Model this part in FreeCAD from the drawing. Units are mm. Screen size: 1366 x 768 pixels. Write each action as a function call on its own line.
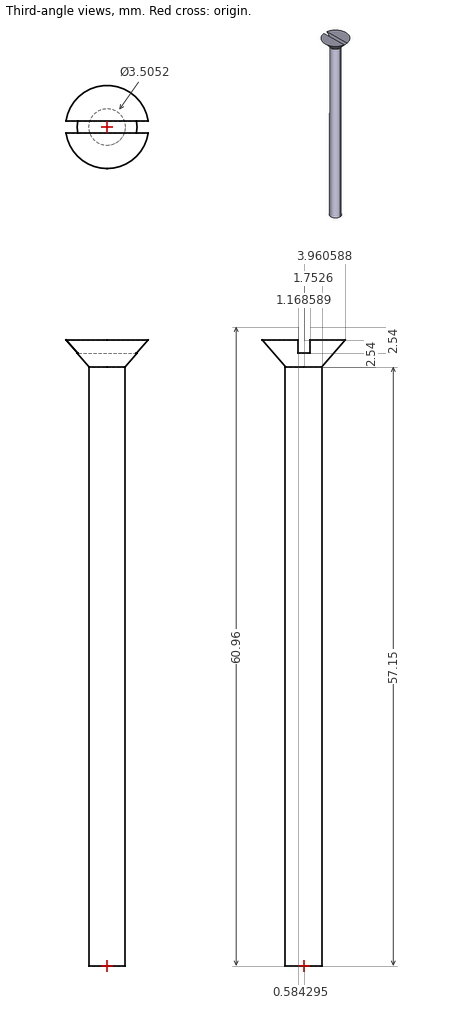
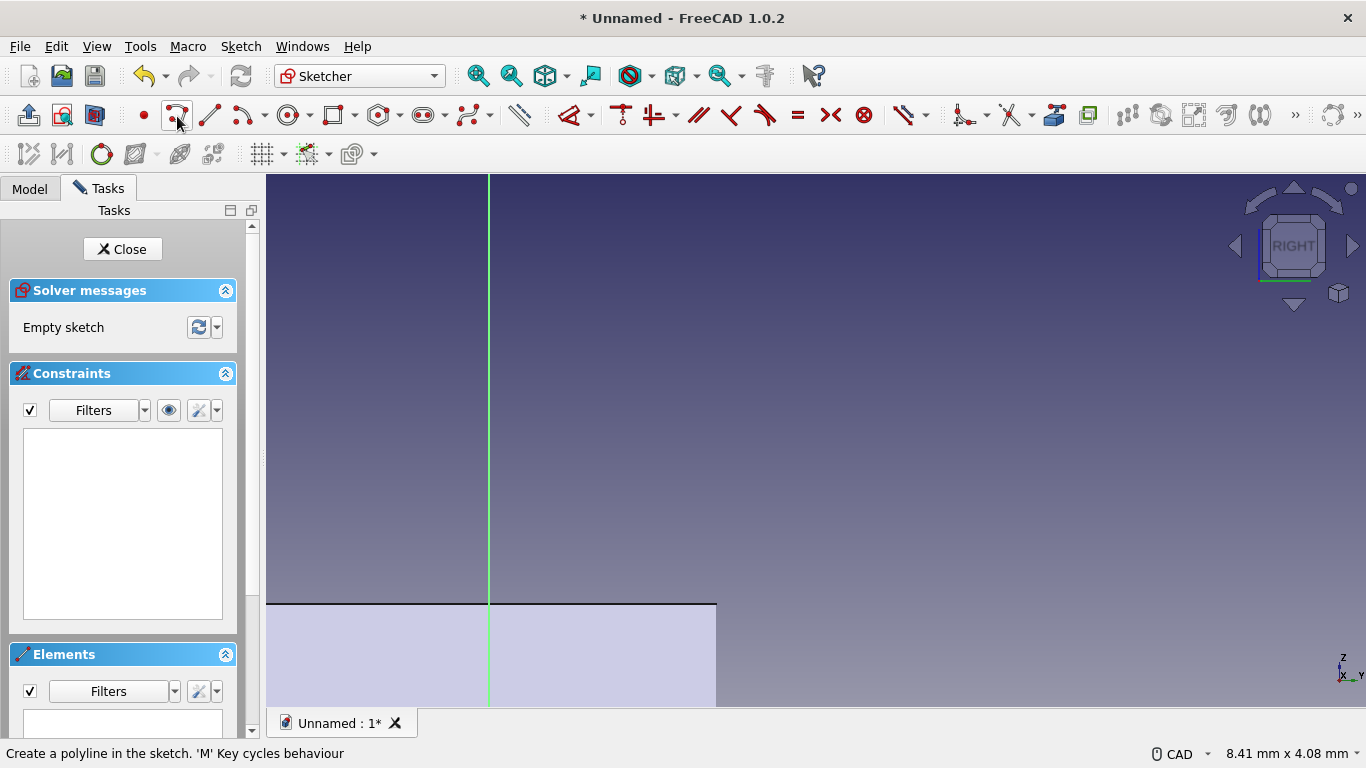
click(489, 604)
click(718, 604)
click(1006, 272)
click(498, 272)
click(489, 605)
key(Escape)
key(Escape)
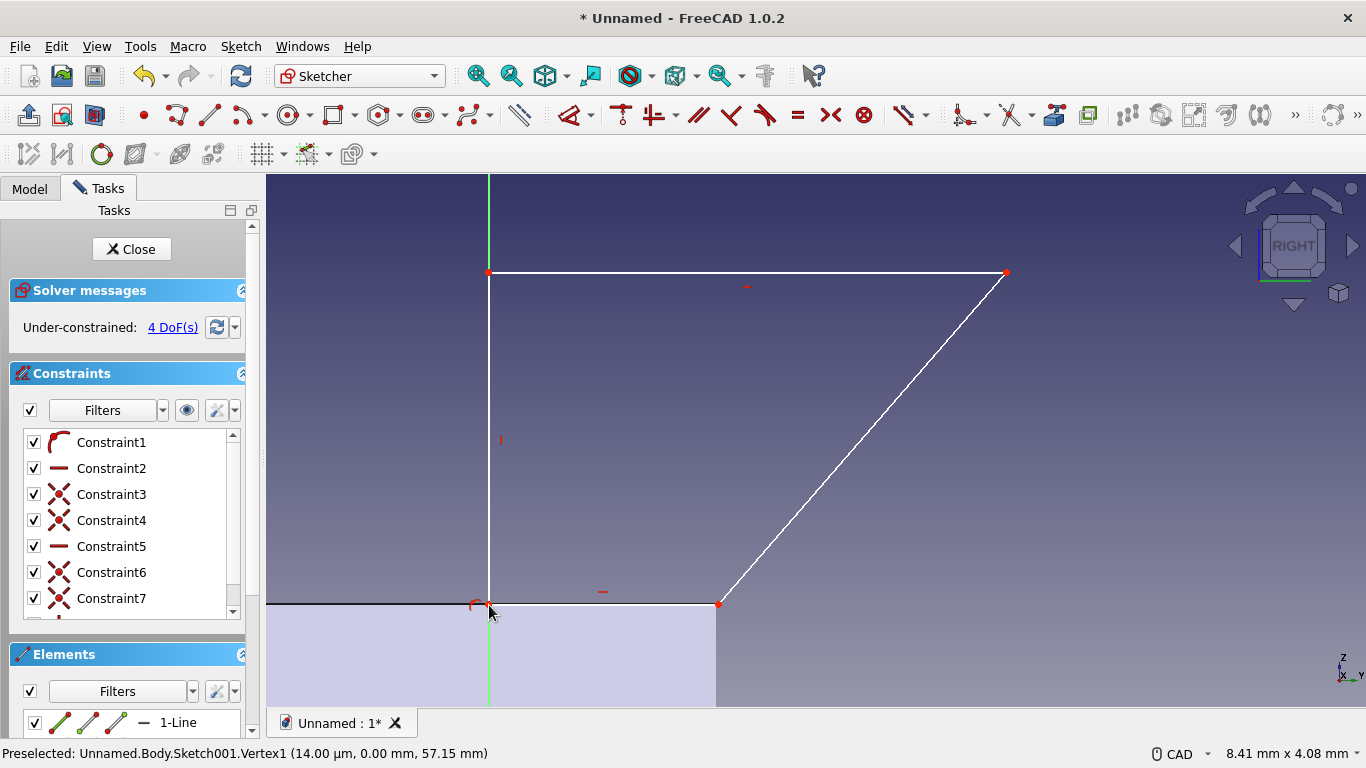
click(568, 116)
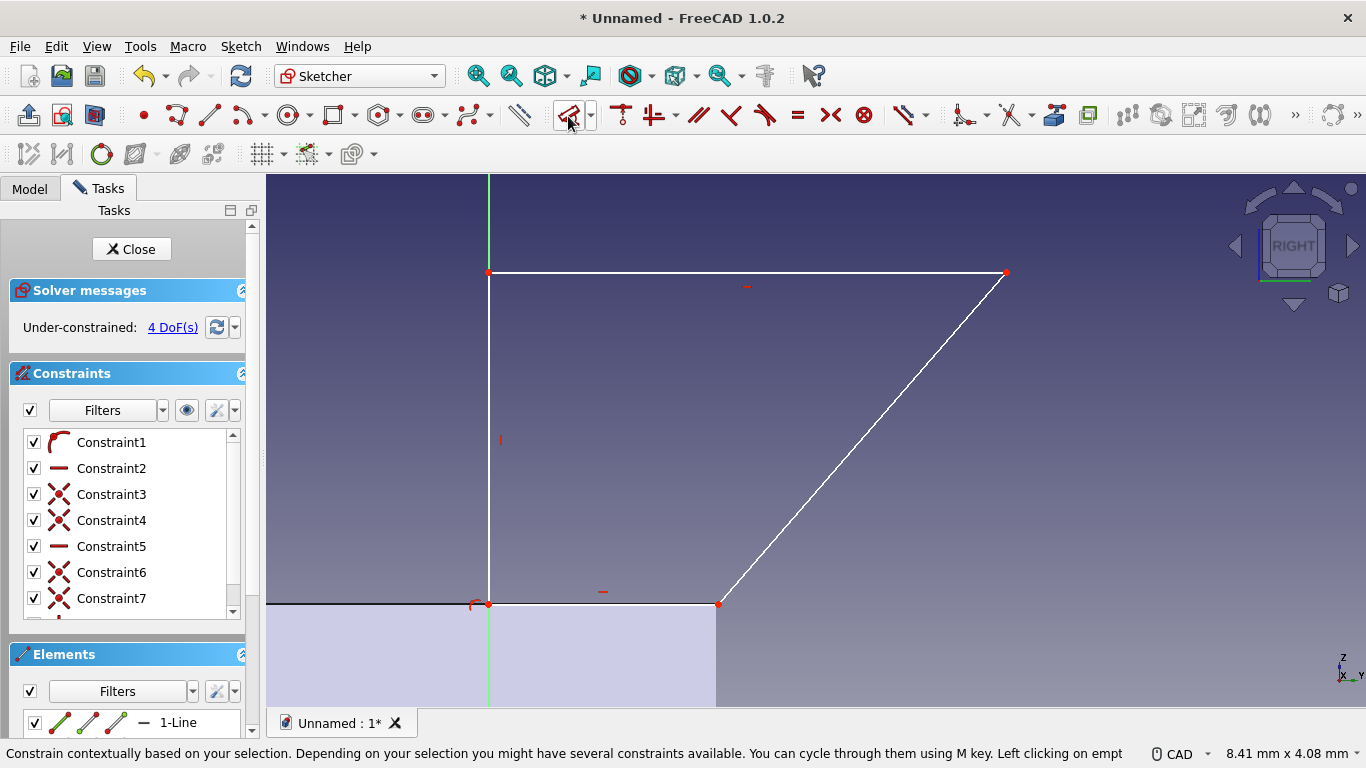
click(489, 373)
click(455, 439)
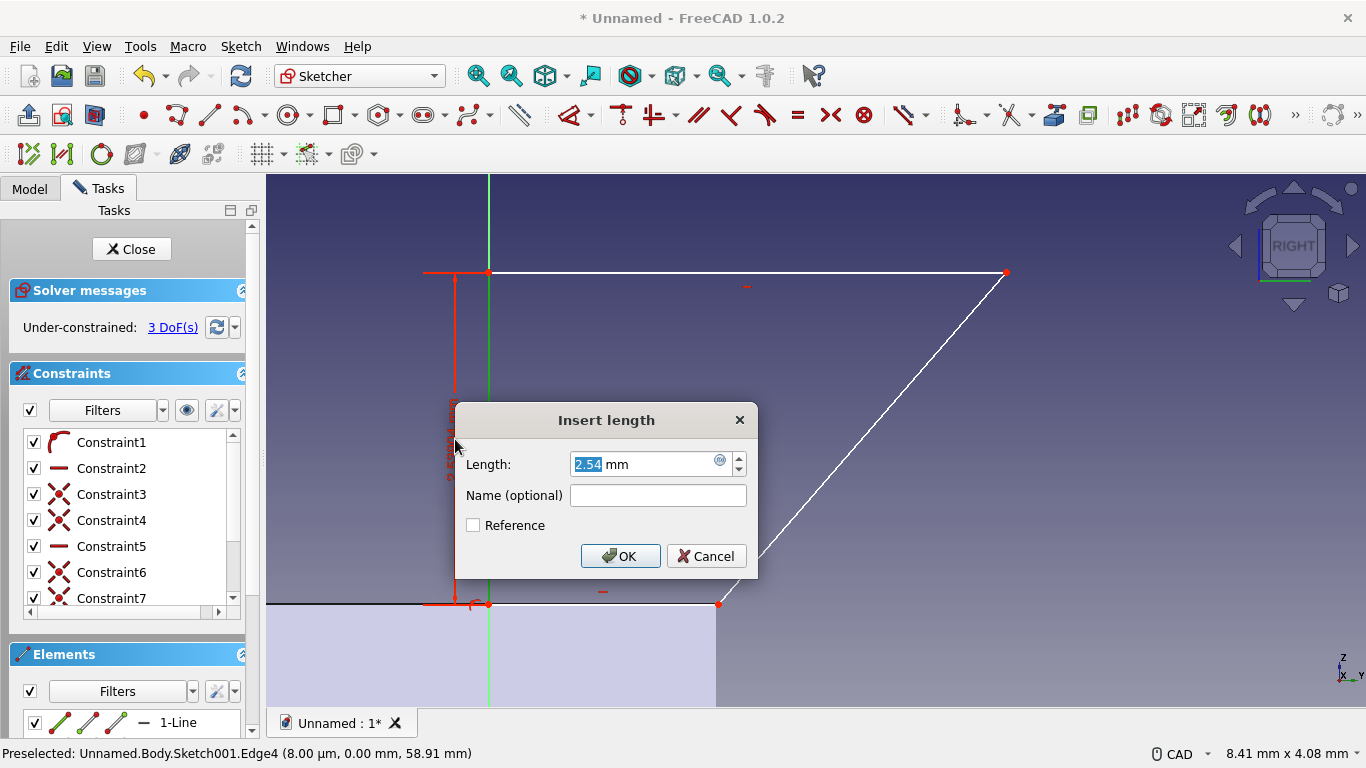
text(2.54)
key(Return)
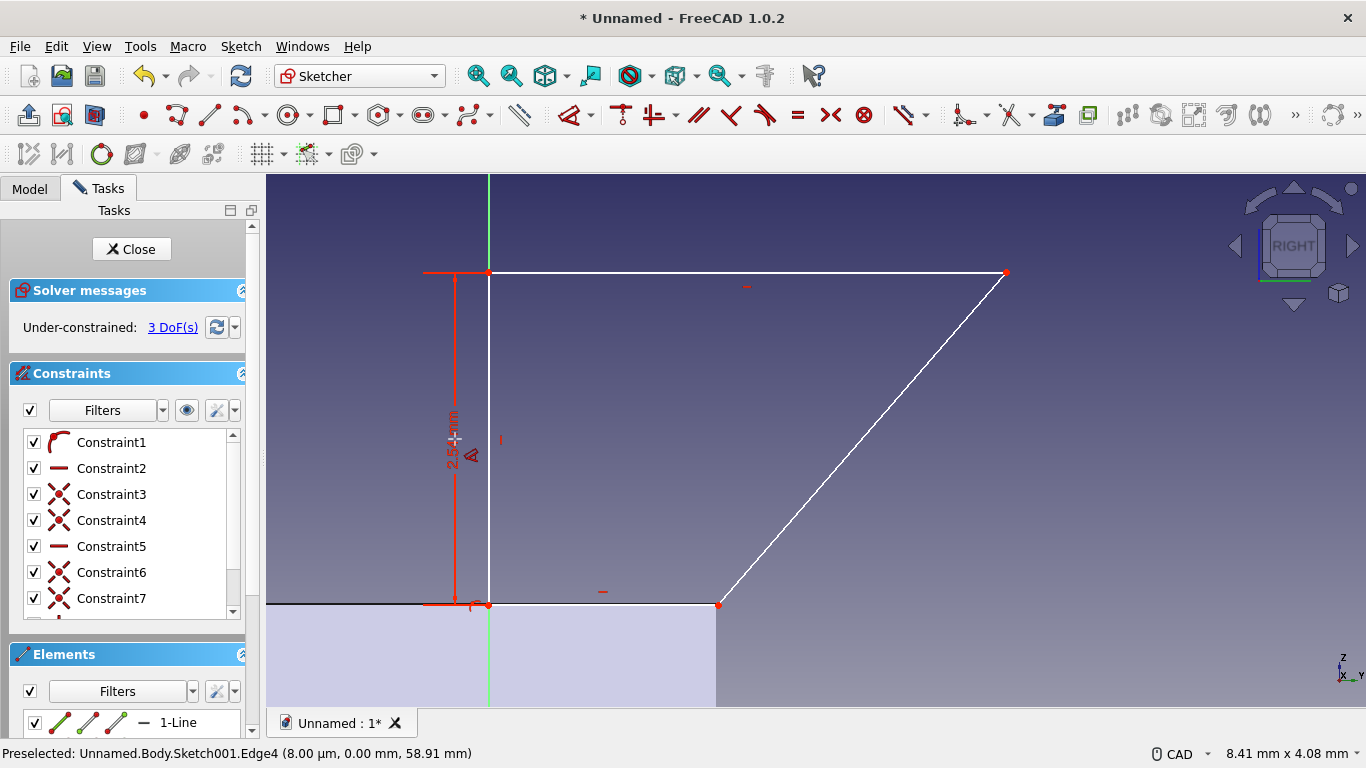
click(557, 605)
click(603, 639)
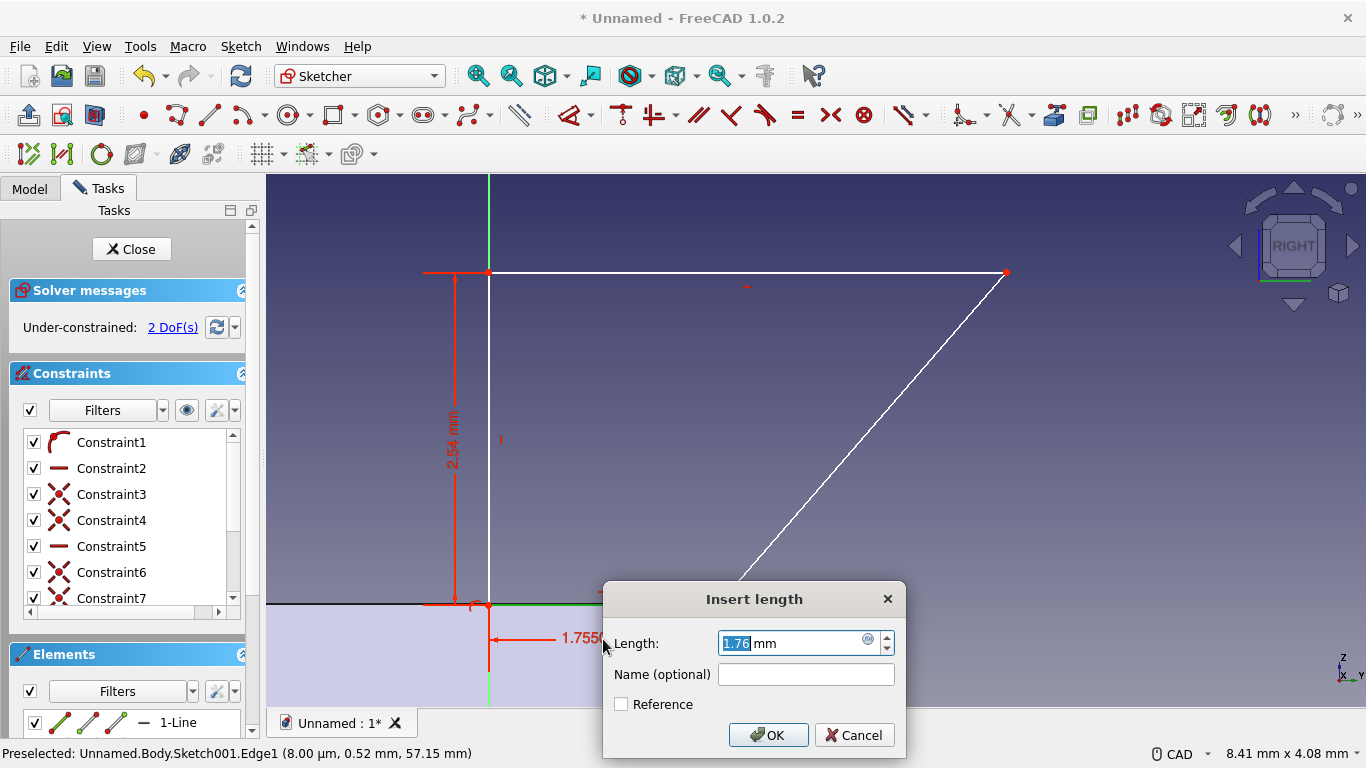
text(1.7526)
key(Return)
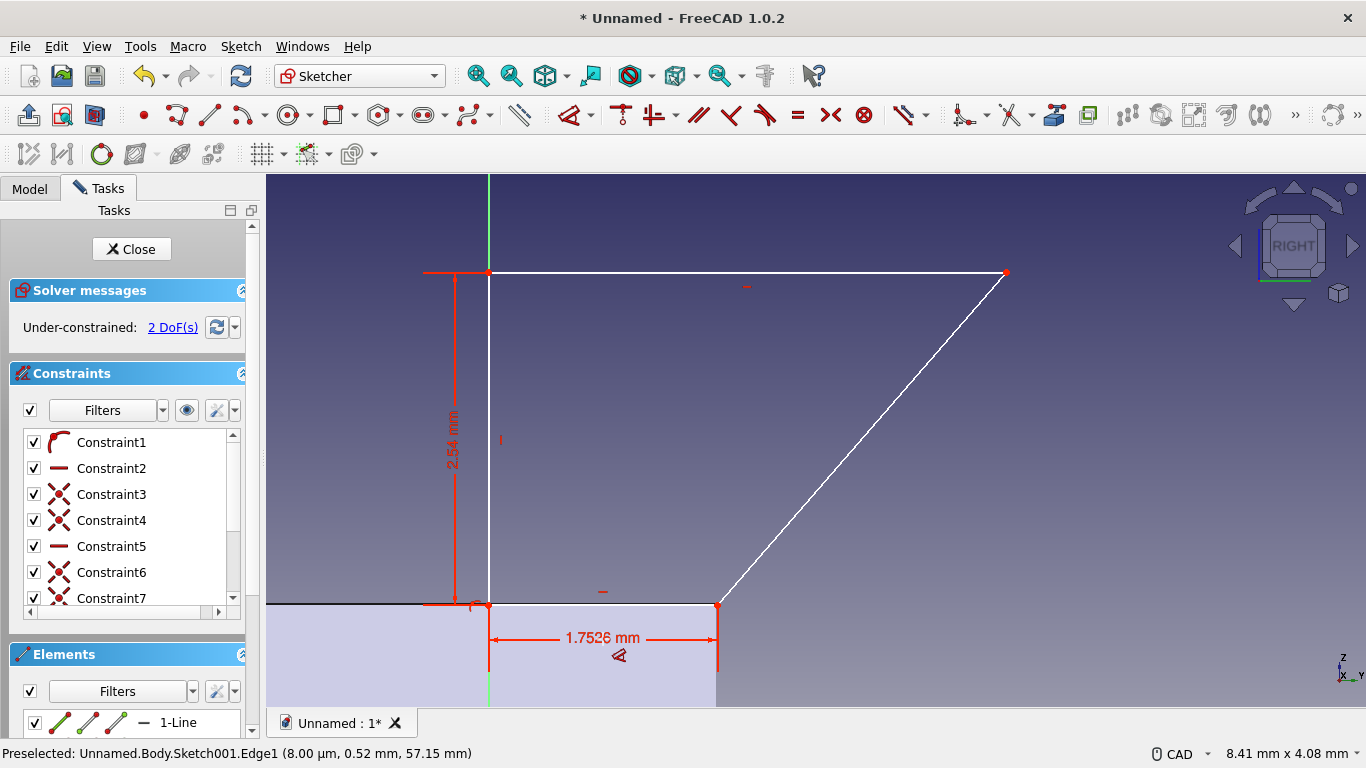
click(489, 605)
click(455, 642)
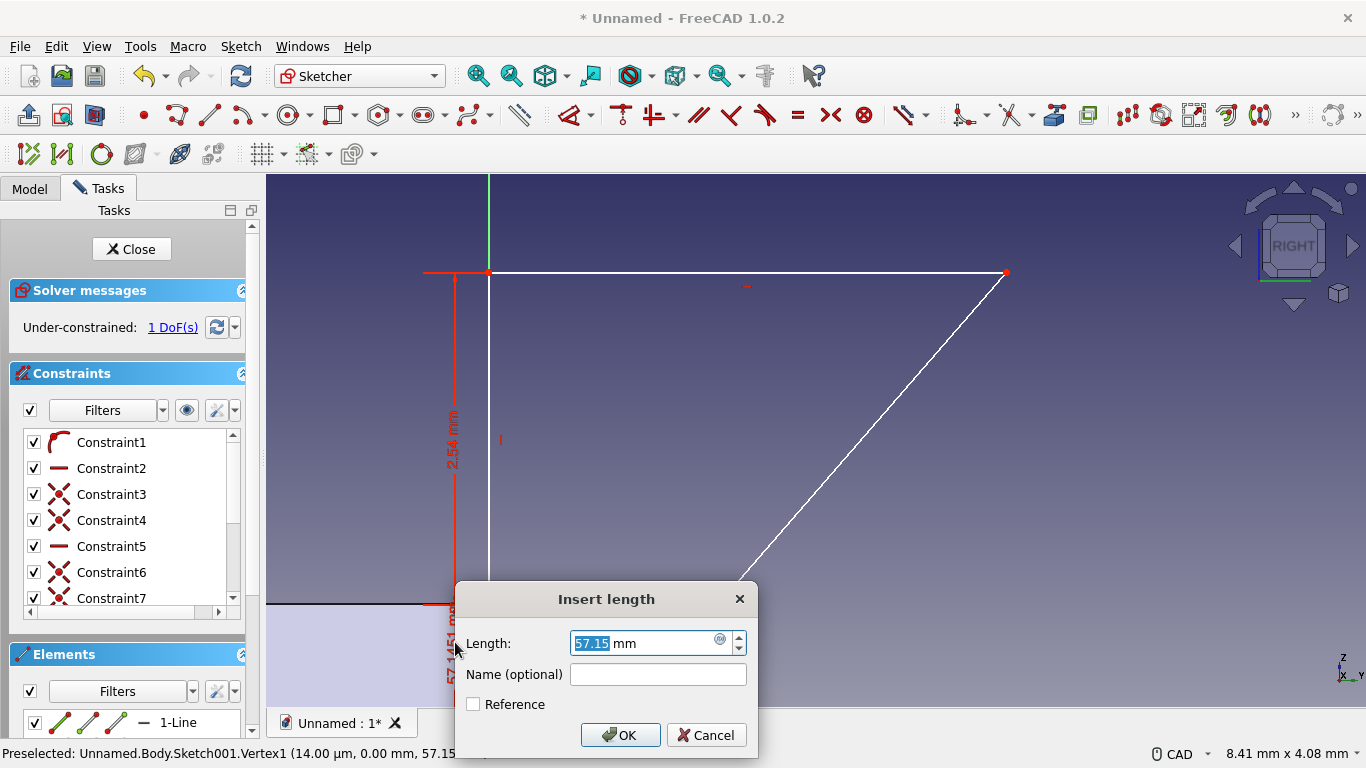
text(57.15)
key(Return)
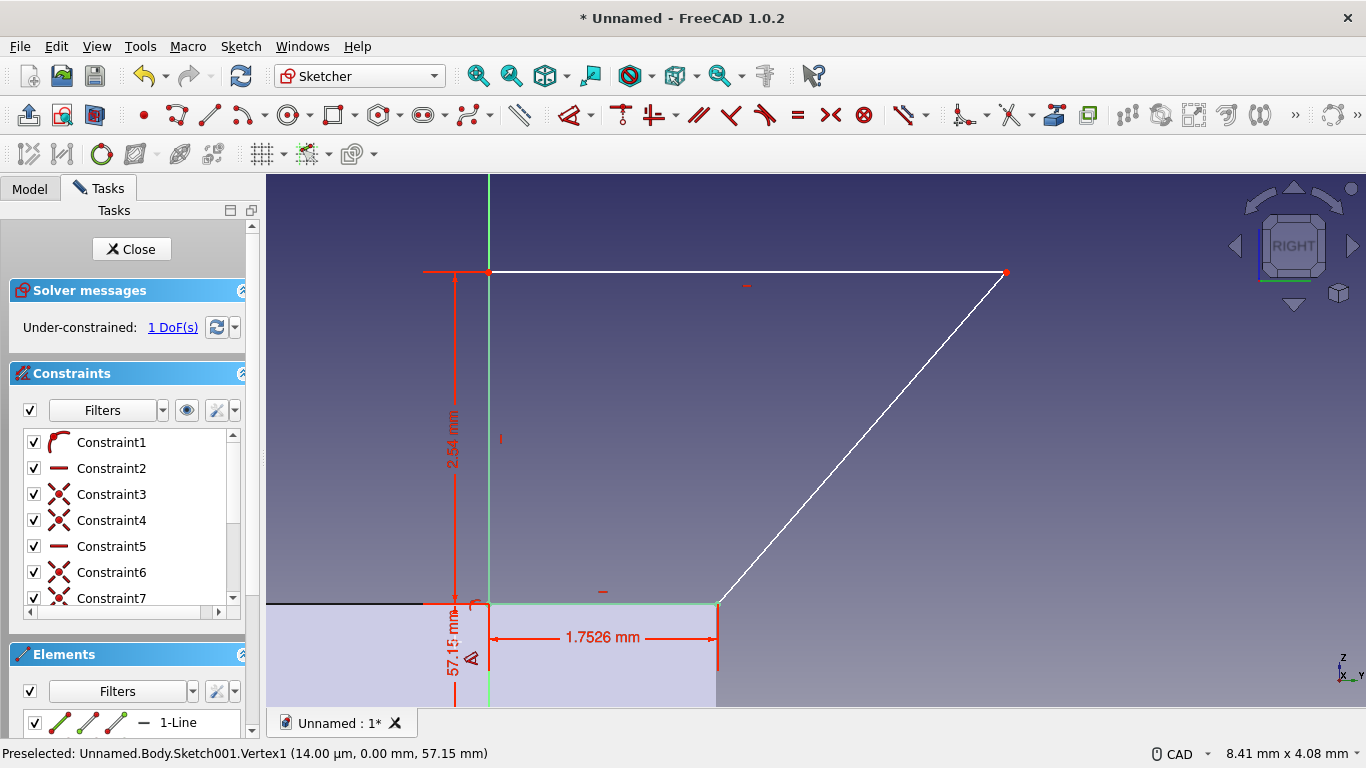
click(851, 272)
click(747, 238)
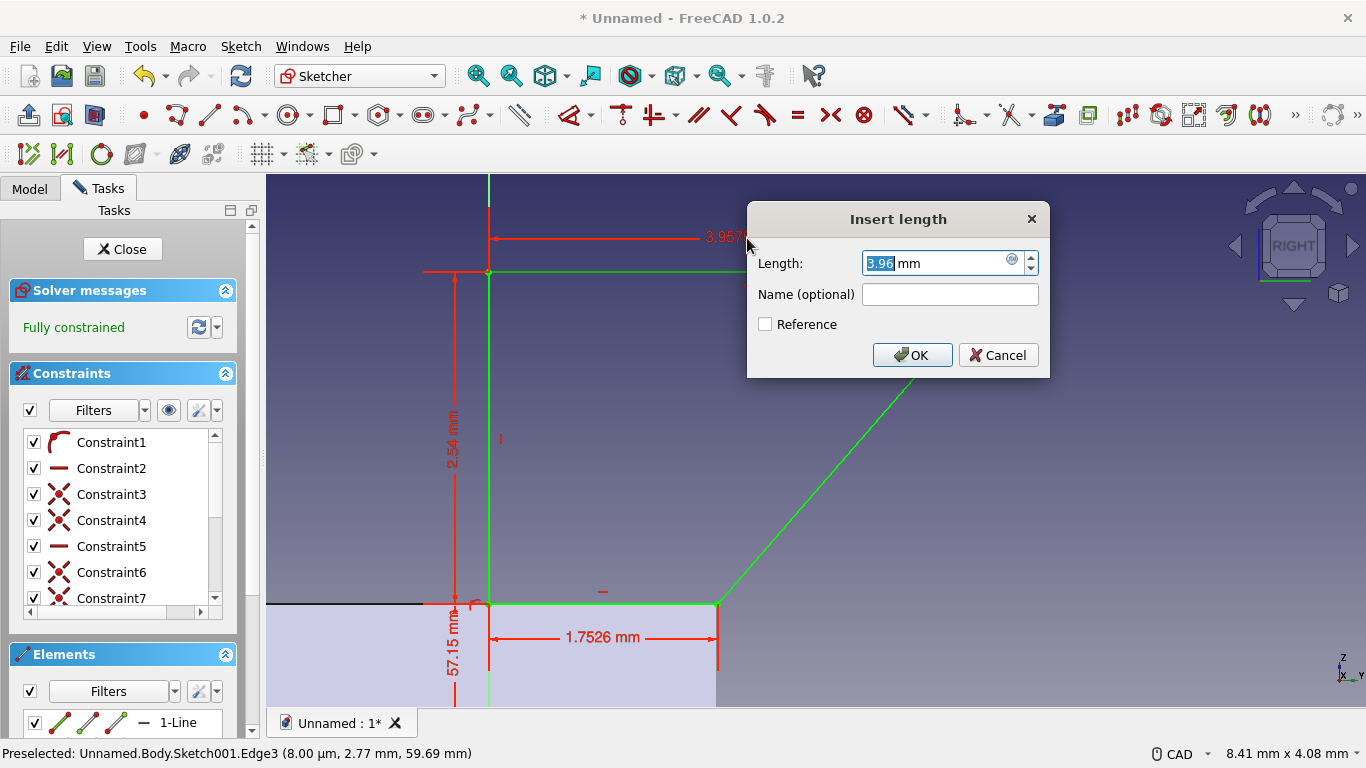
text(3.960588)
key(Return)
key(Escape)